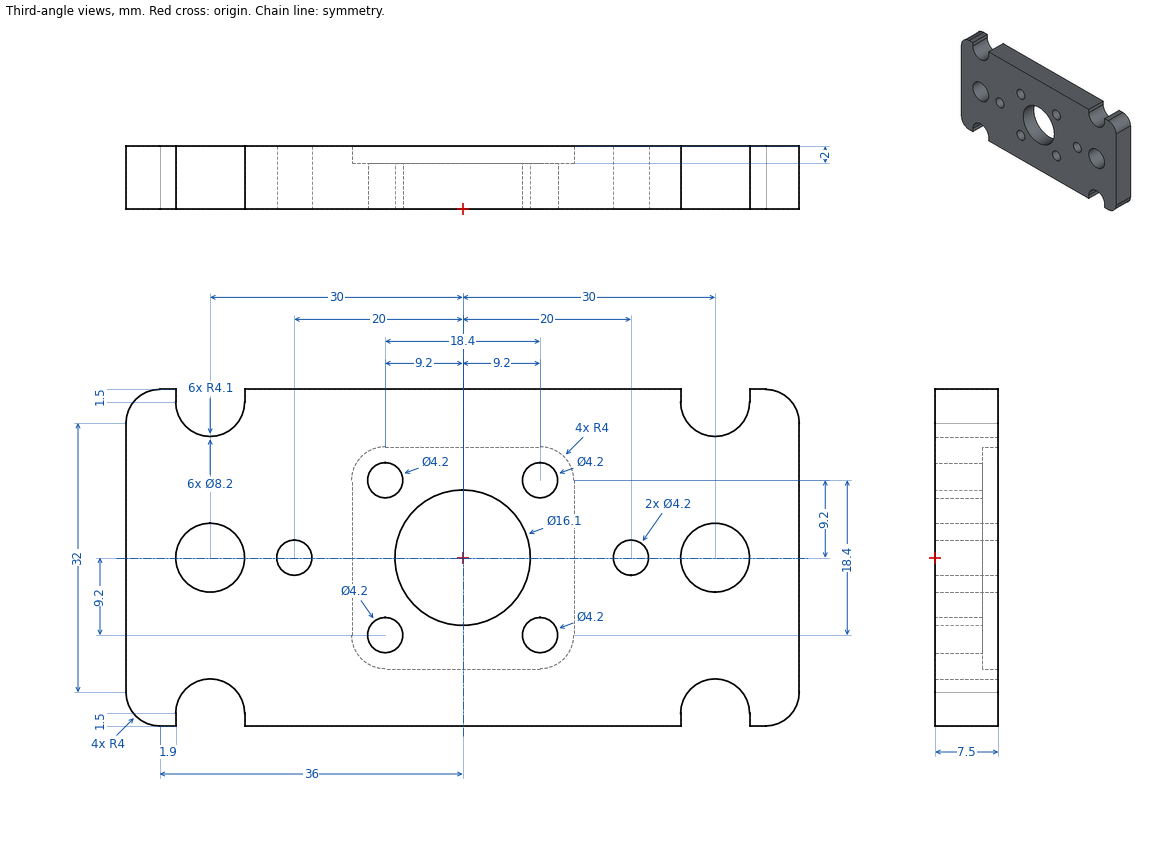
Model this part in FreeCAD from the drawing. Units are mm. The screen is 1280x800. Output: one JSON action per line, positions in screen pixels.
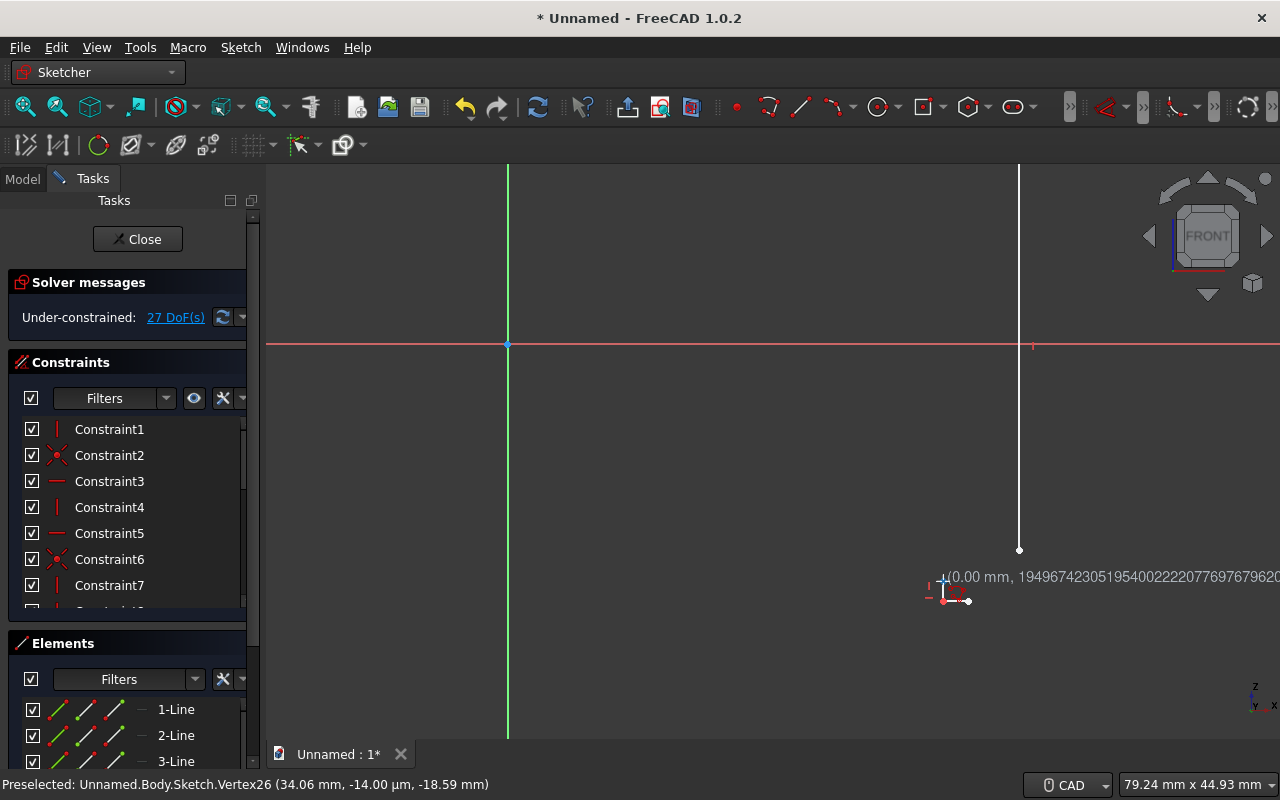
{"action": "left_click", "coordinate": [839, 581]}
{"action": "left_click", "coordinate": [839, 600]}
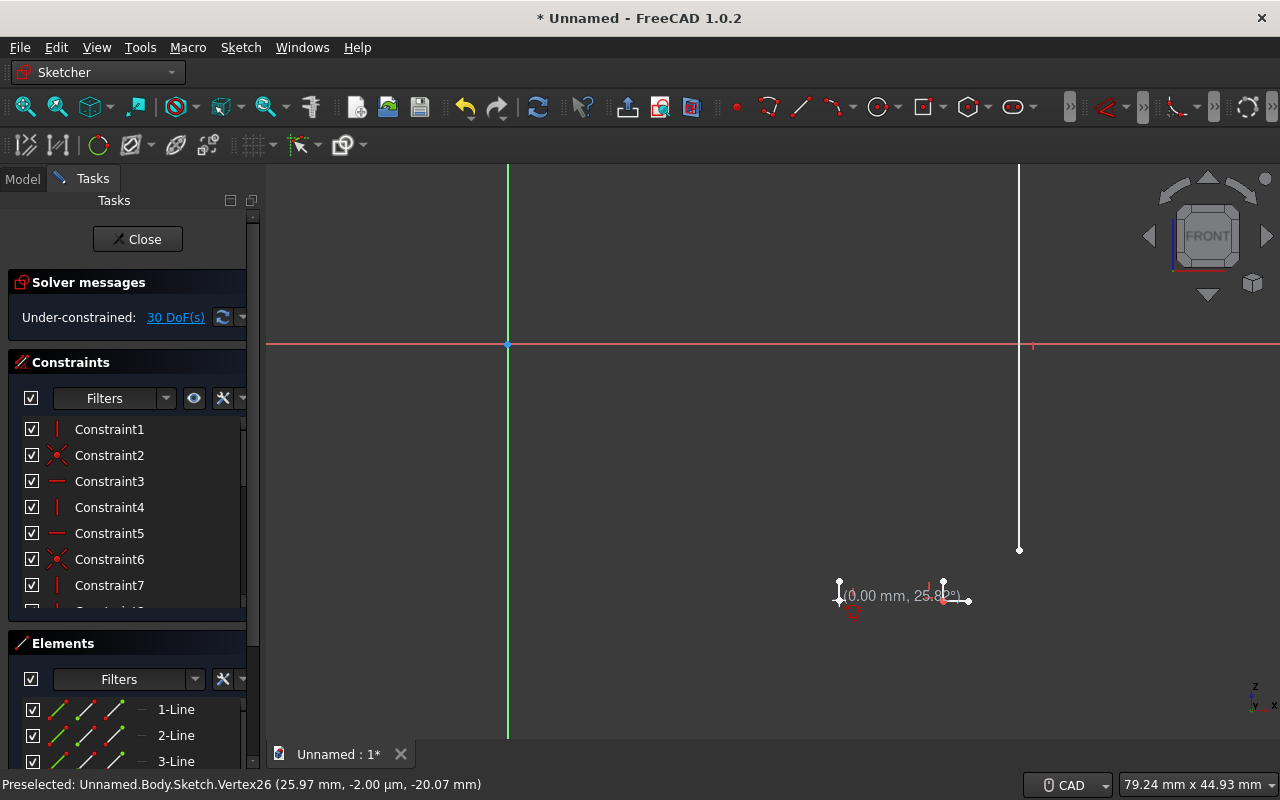
{"action": "scroll", "coordinate": [944, 582], "scroll_direction": "down", "scroll_amount": 3}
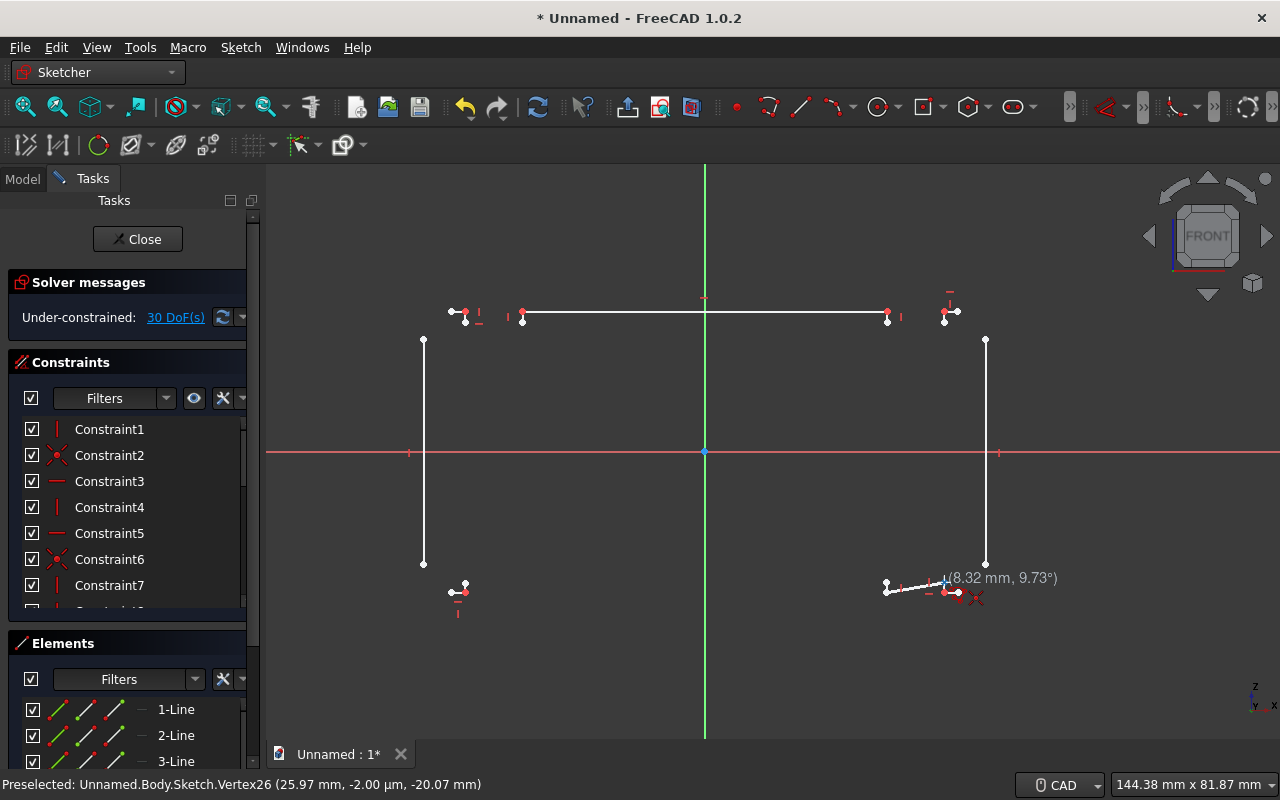
{"action": "left_click", "coordinate": [523, 592]}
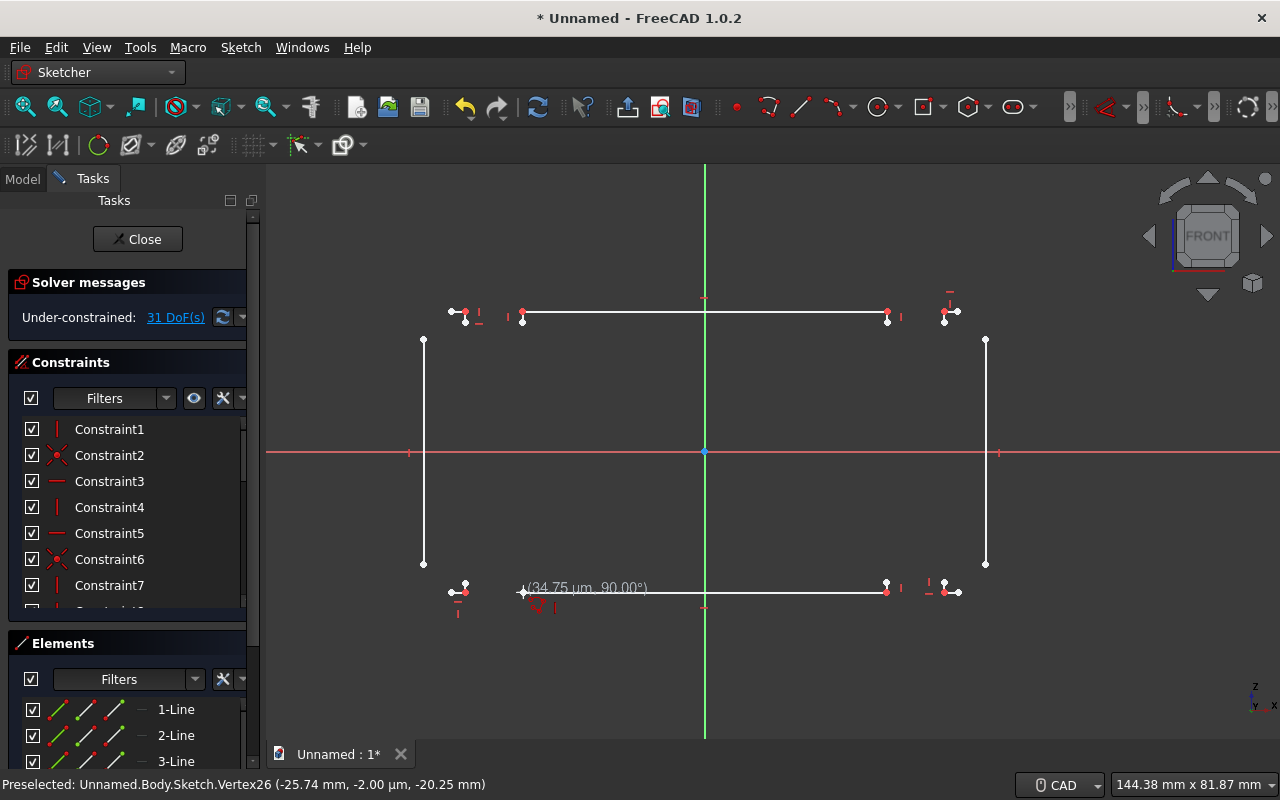
{"action": "scroll", "coordinate": [523, 582], "scroll_direction": "up", "scroll_amount": 3}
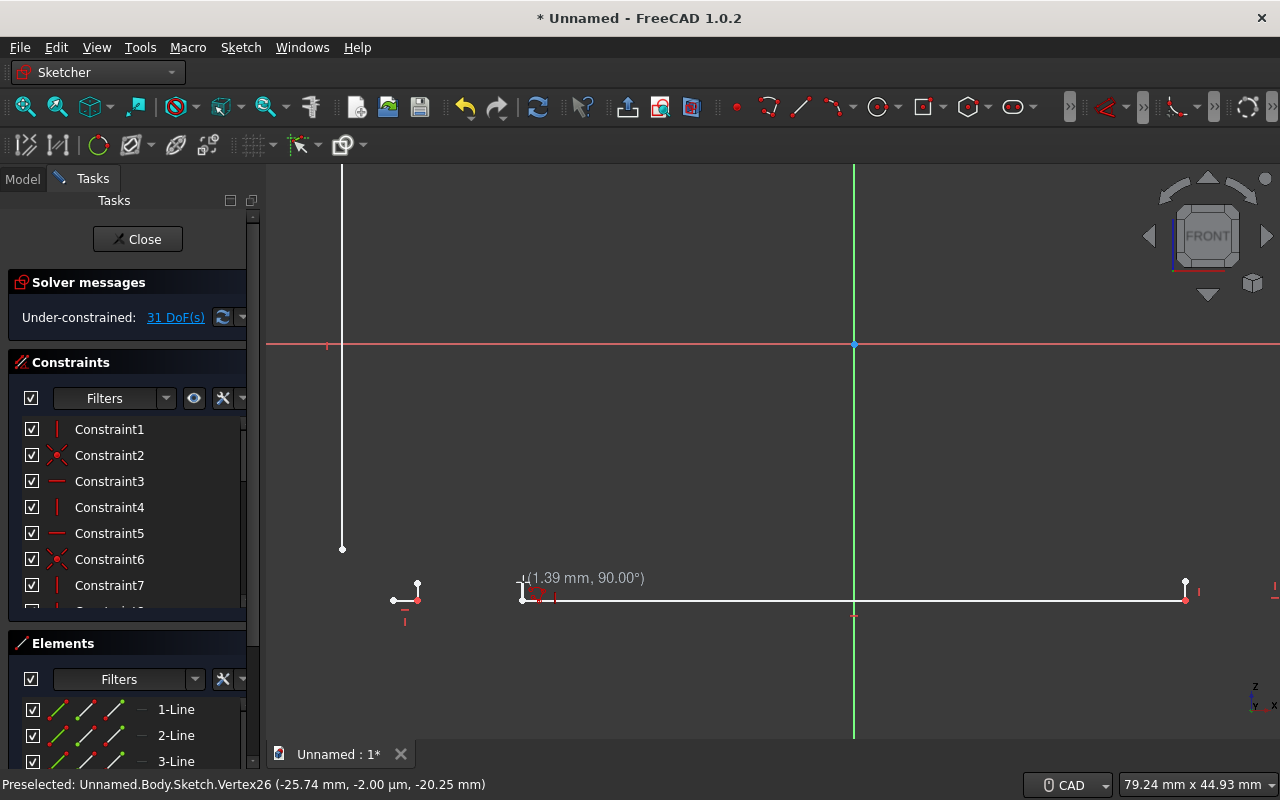
{"action": "left_click", "coordinate": [523, 581]}
{"action": "right_click", "coordinate": [523, 581]}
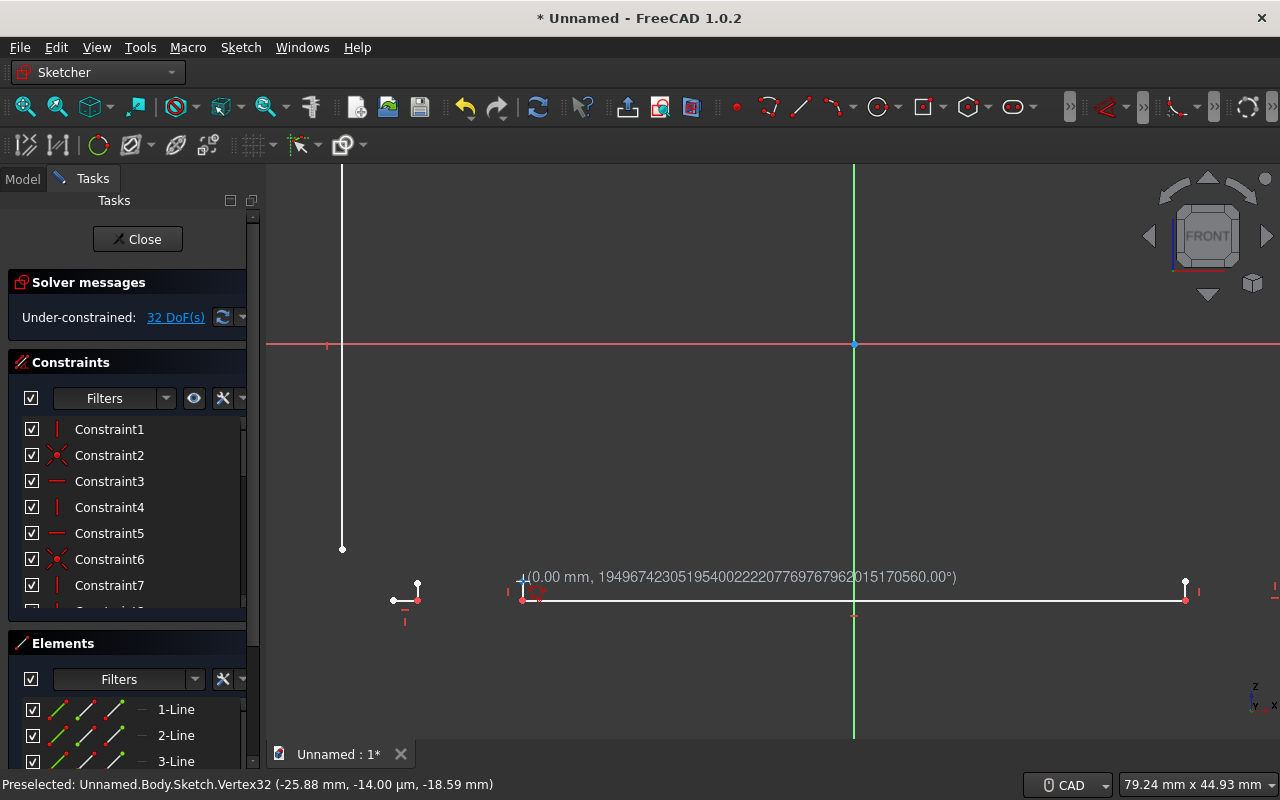
{"action": "left_click", "coordinate": [834, 108]}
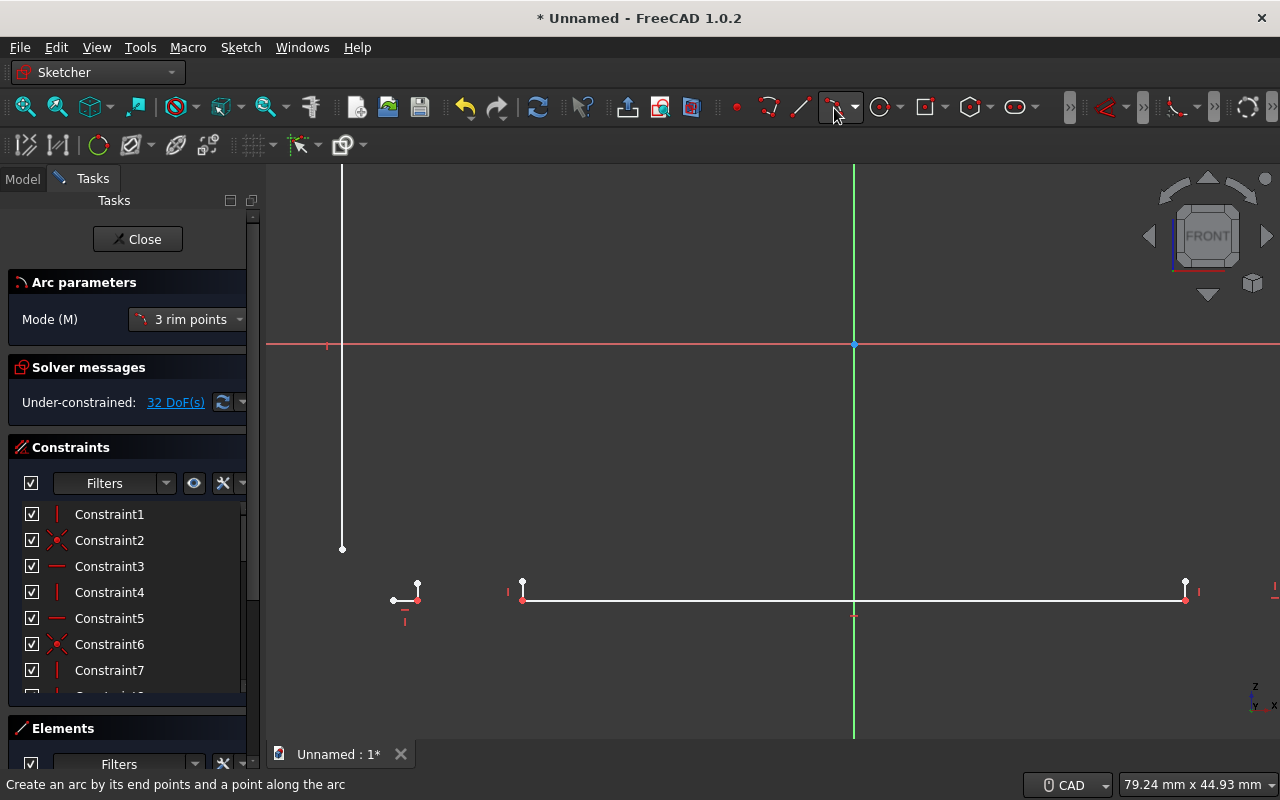
{"action": "scroll", "coordinate": [393, 600], "scroll_direction": "up", "scroll_amount": 2}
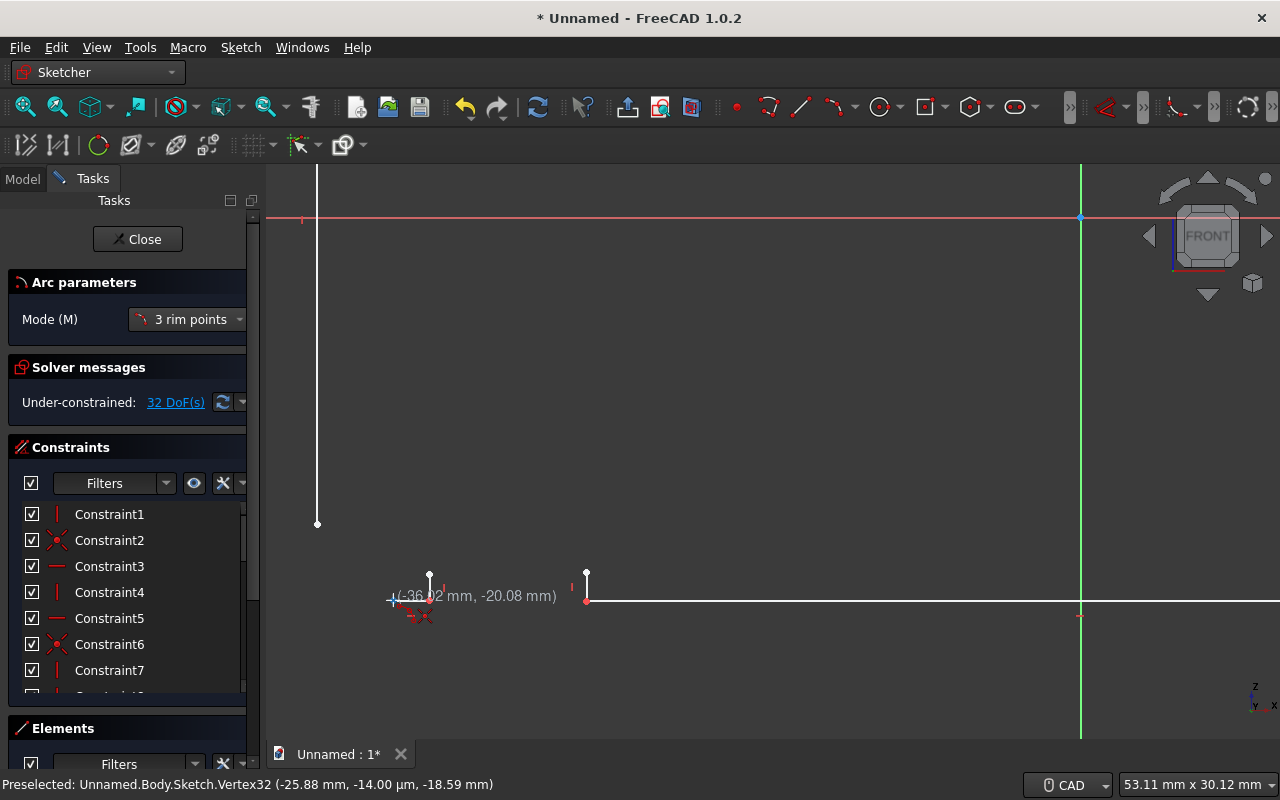
{"action": "left_click", "coordinate": [393, 601]}
{"action": "left_click", "coordinate": [317, 525]}
{"action": "left_click", "coordinate": [339, 577]}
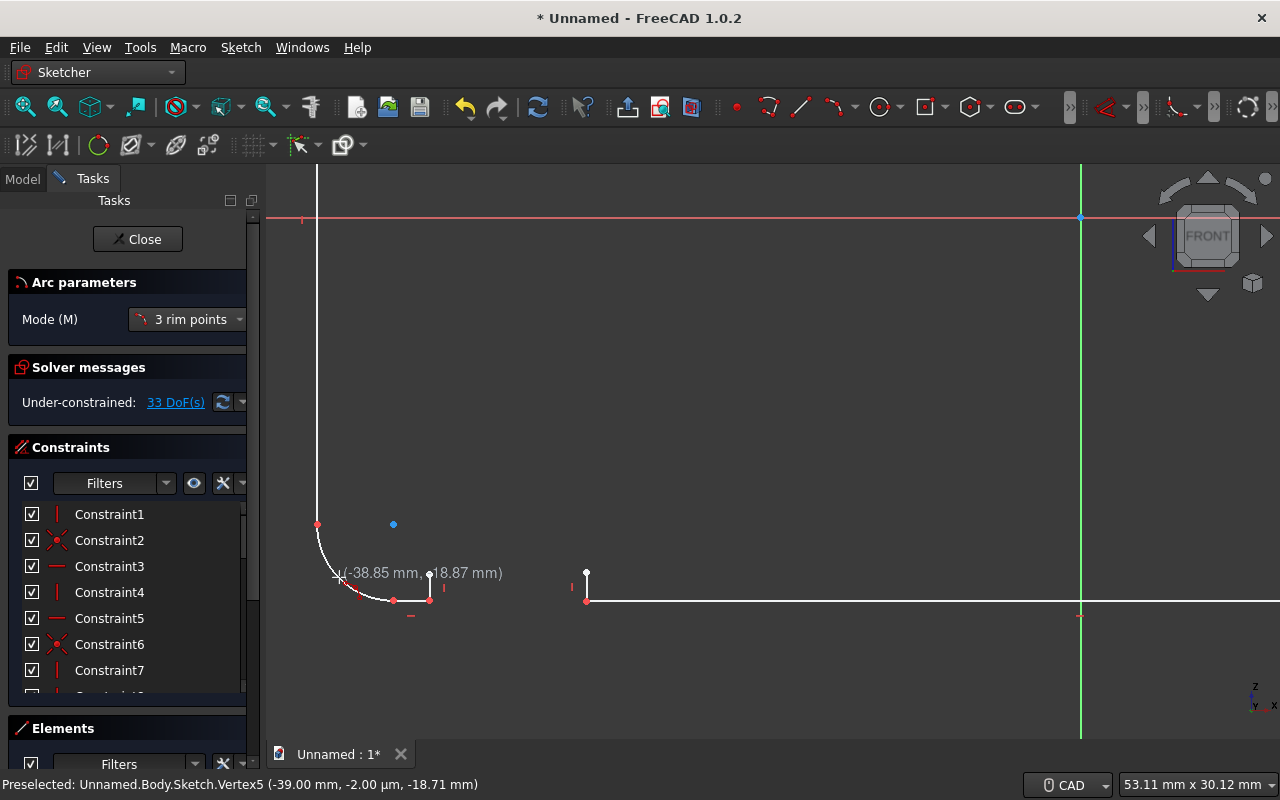
{"action": "scroll", "coordinate": [486, 587], "scroll_direction": "down", "scroll_amount": 5}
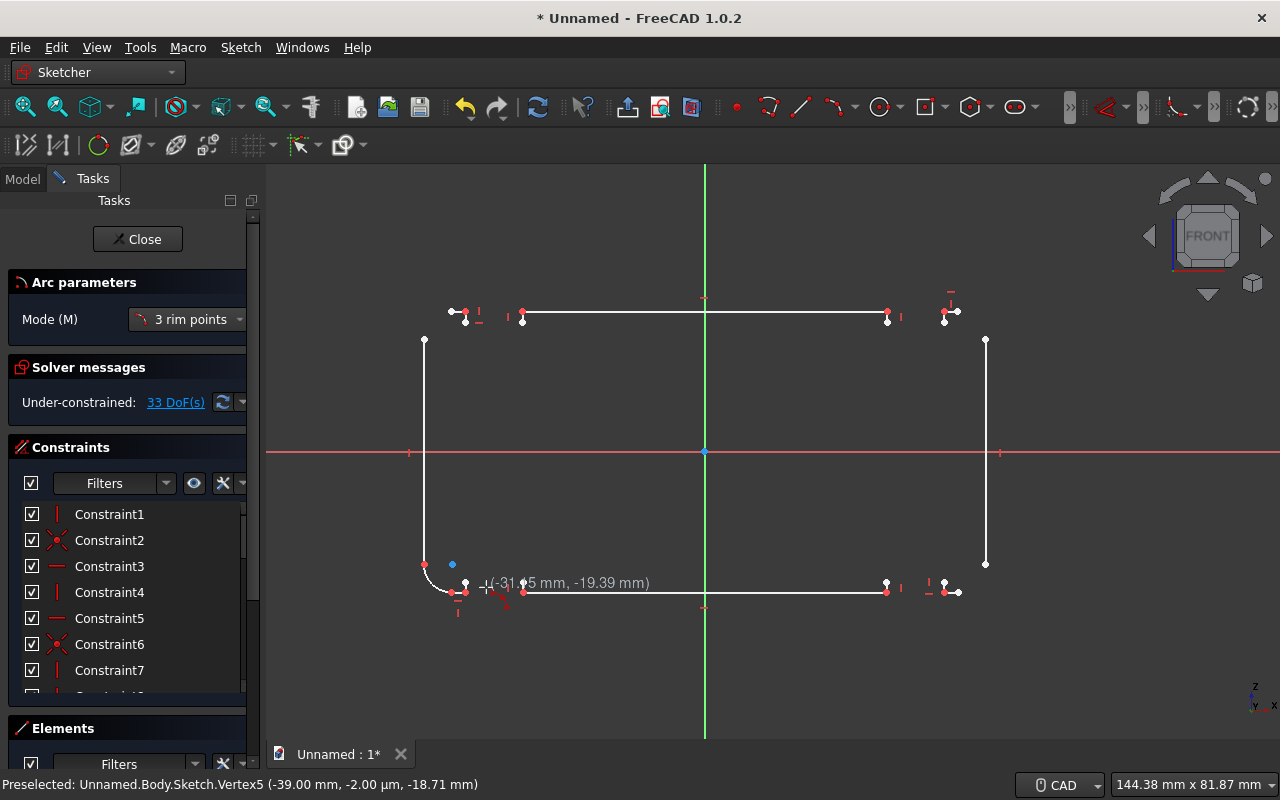
{"action": "left_click", "coordinate": [424, 340]}